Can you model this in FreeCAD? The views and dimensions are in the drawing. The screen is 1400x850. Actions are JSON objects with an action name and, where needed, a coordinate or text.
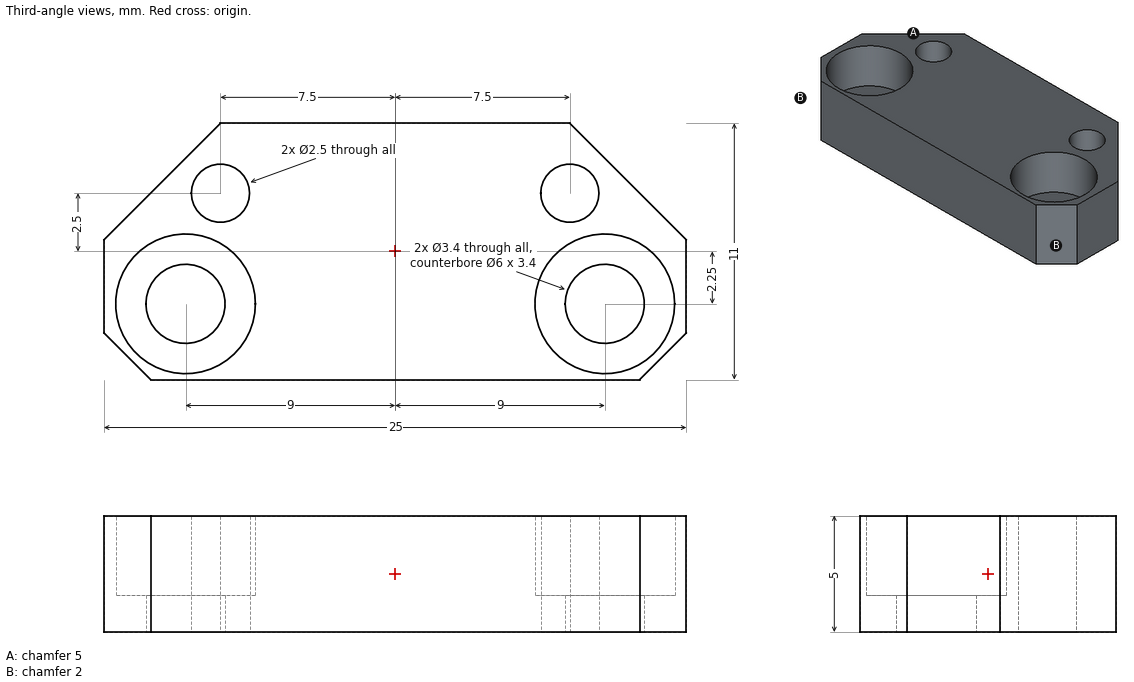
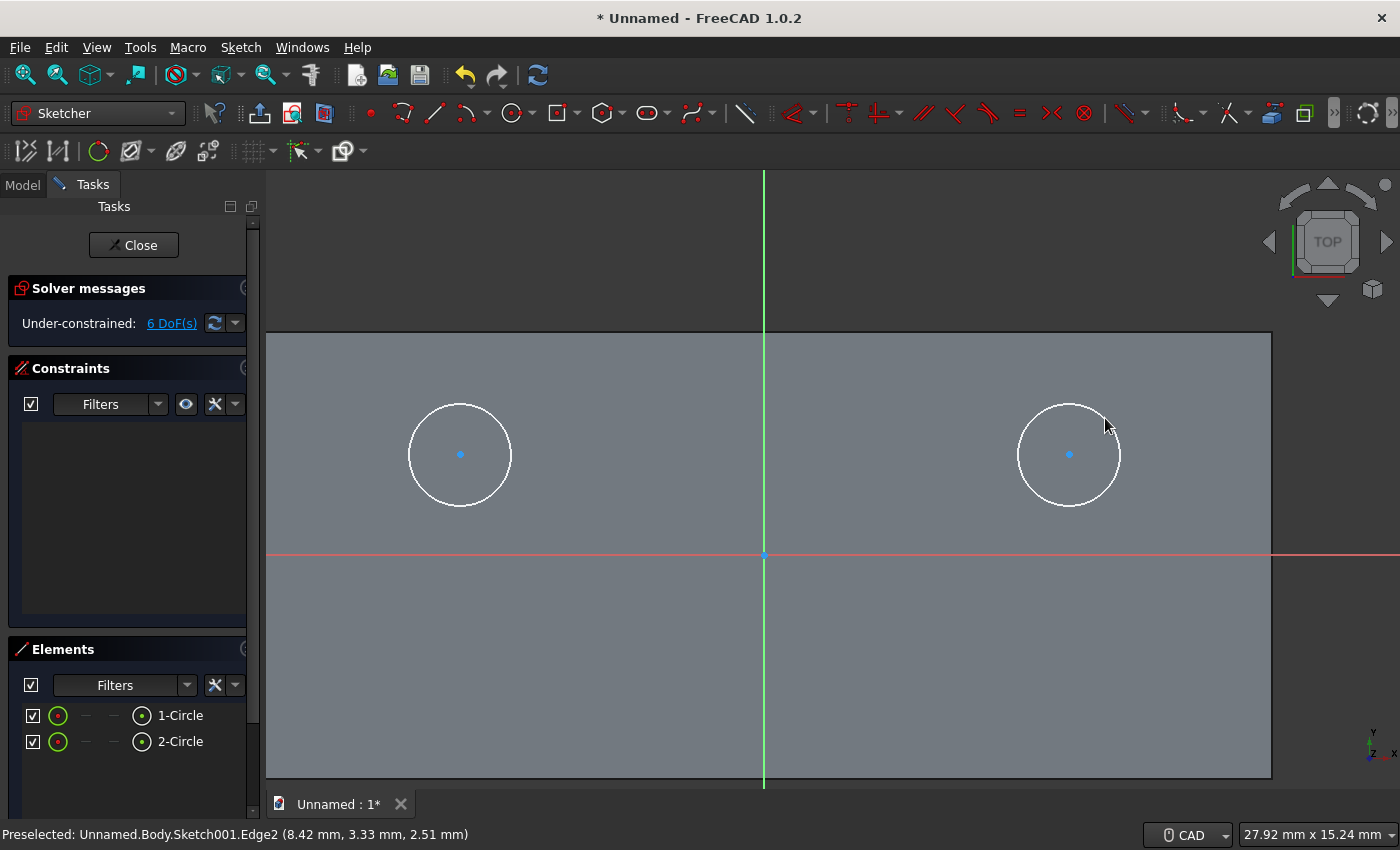
{"action": "left_click", "coordinate": [496, 419]}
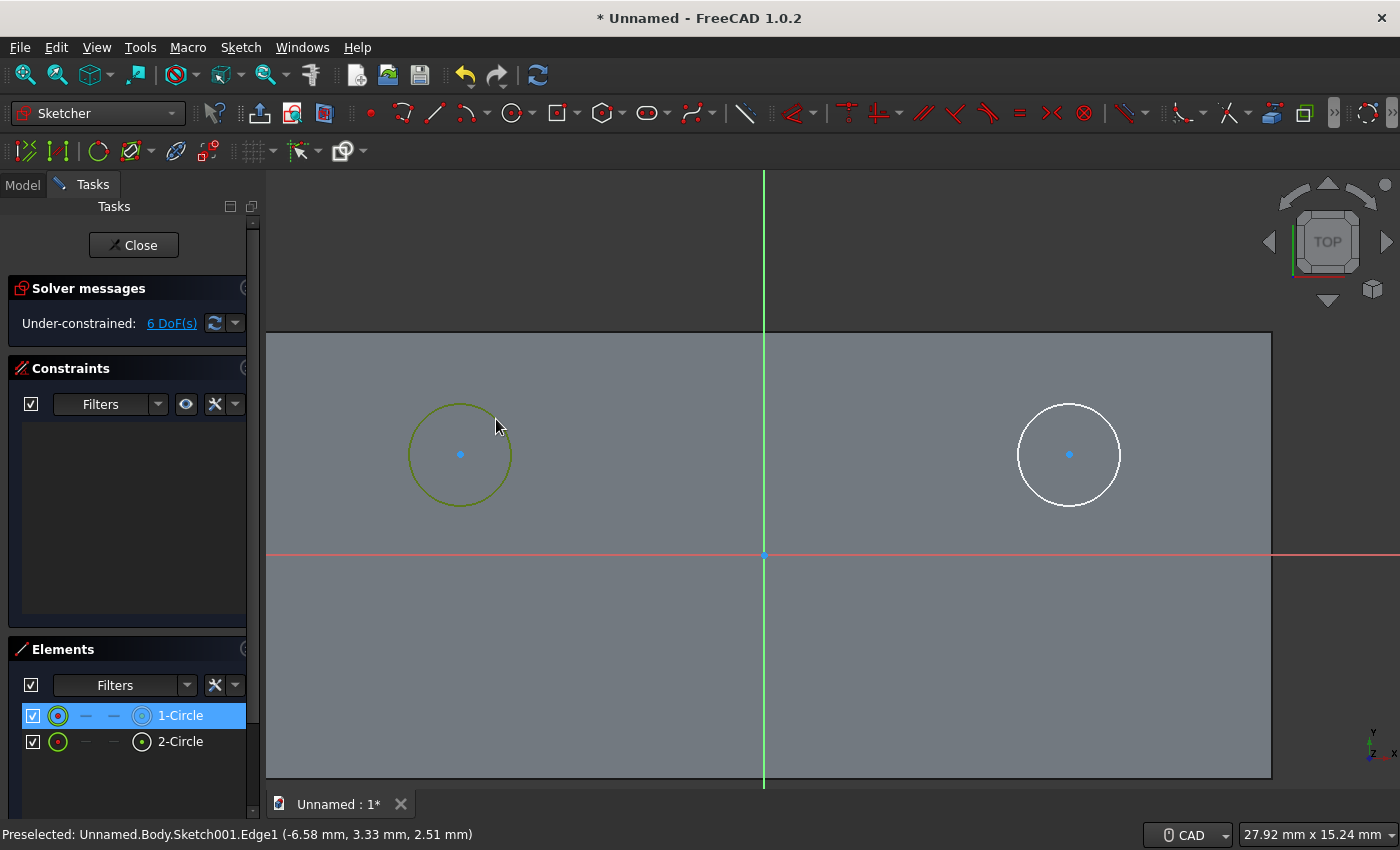
{"action": "left_click", "coordinate": [1105, 419]}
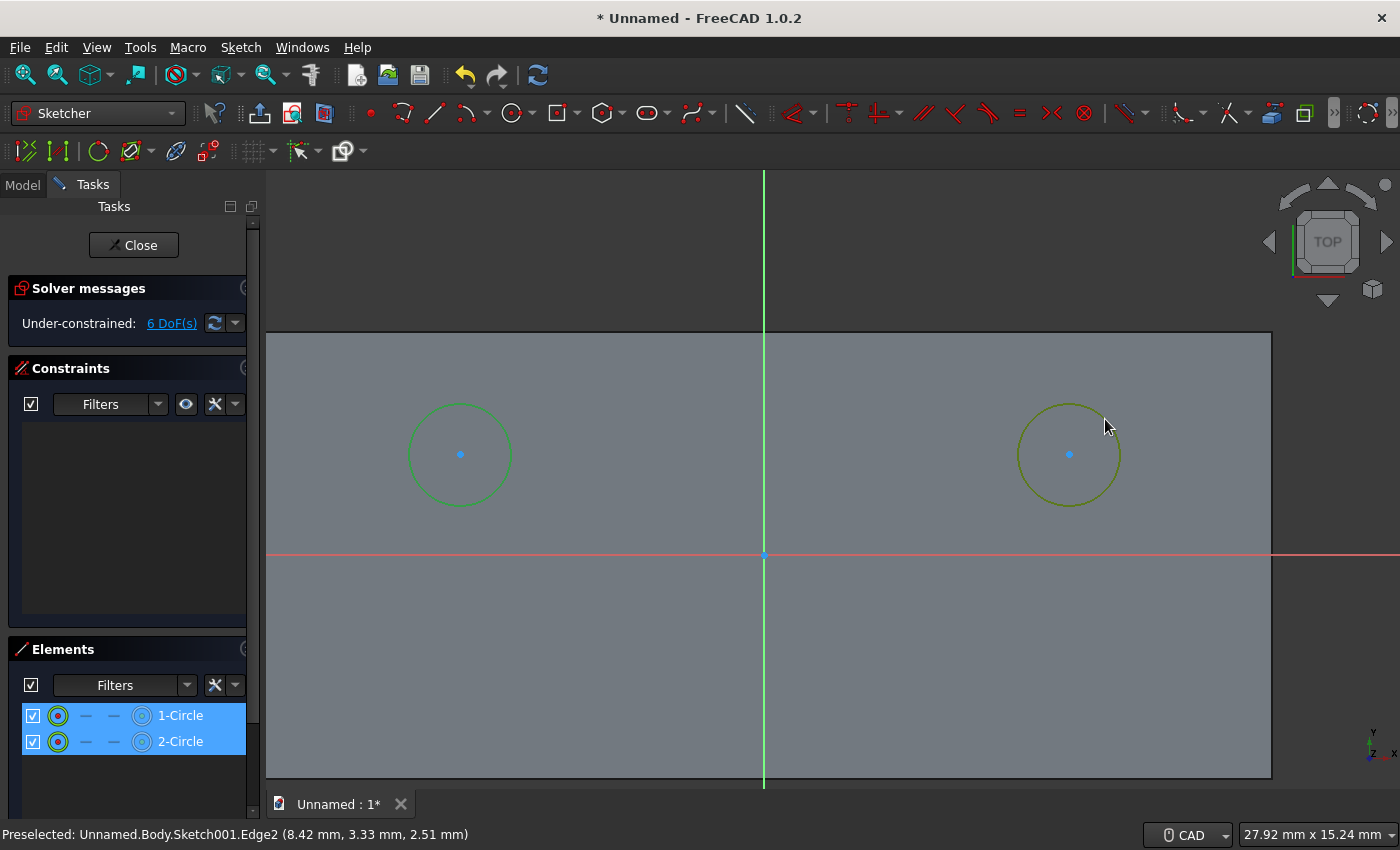
{"action": "key", "text": "e"}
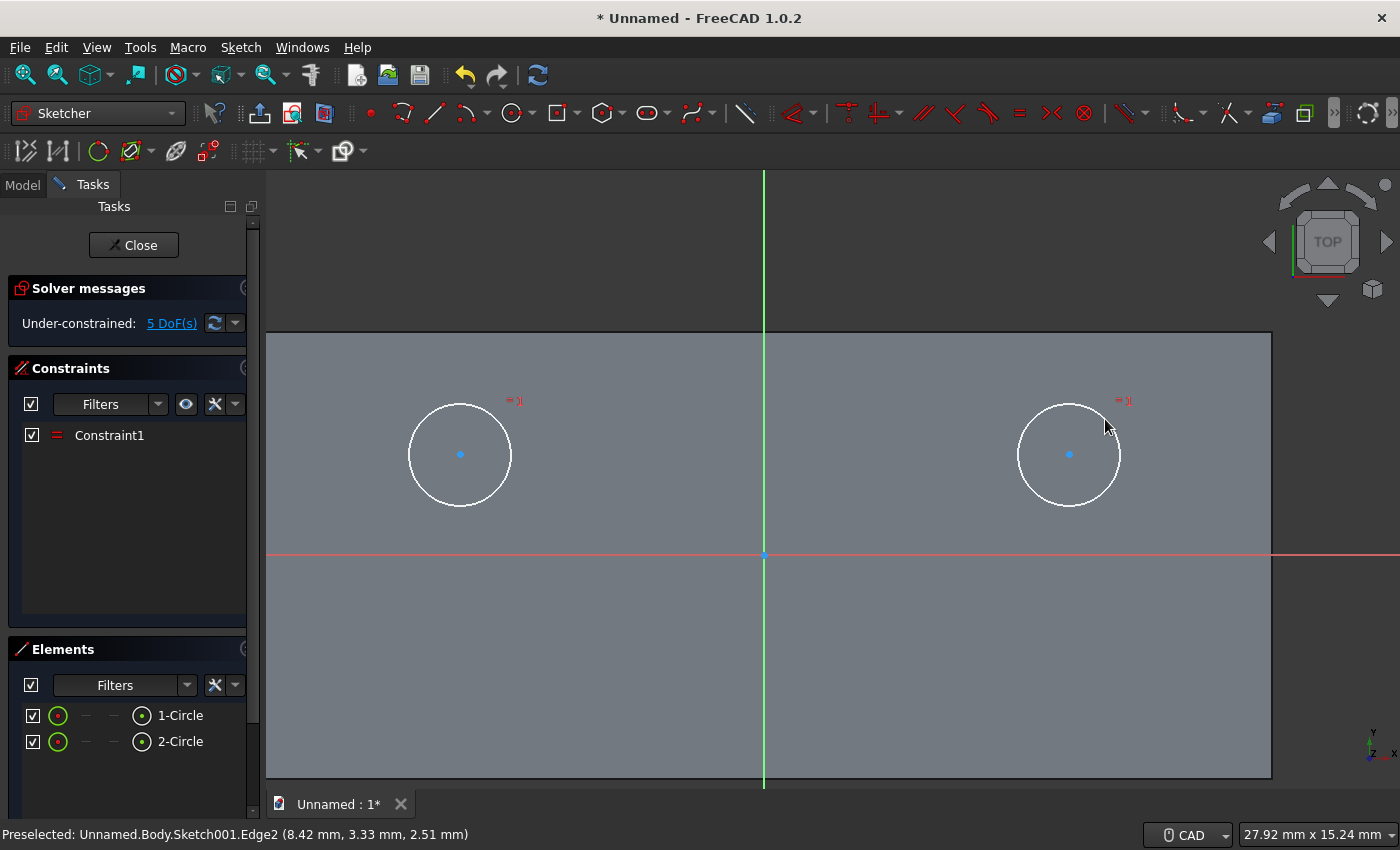
{"action": "left_click", "coordinate": [460, 455]}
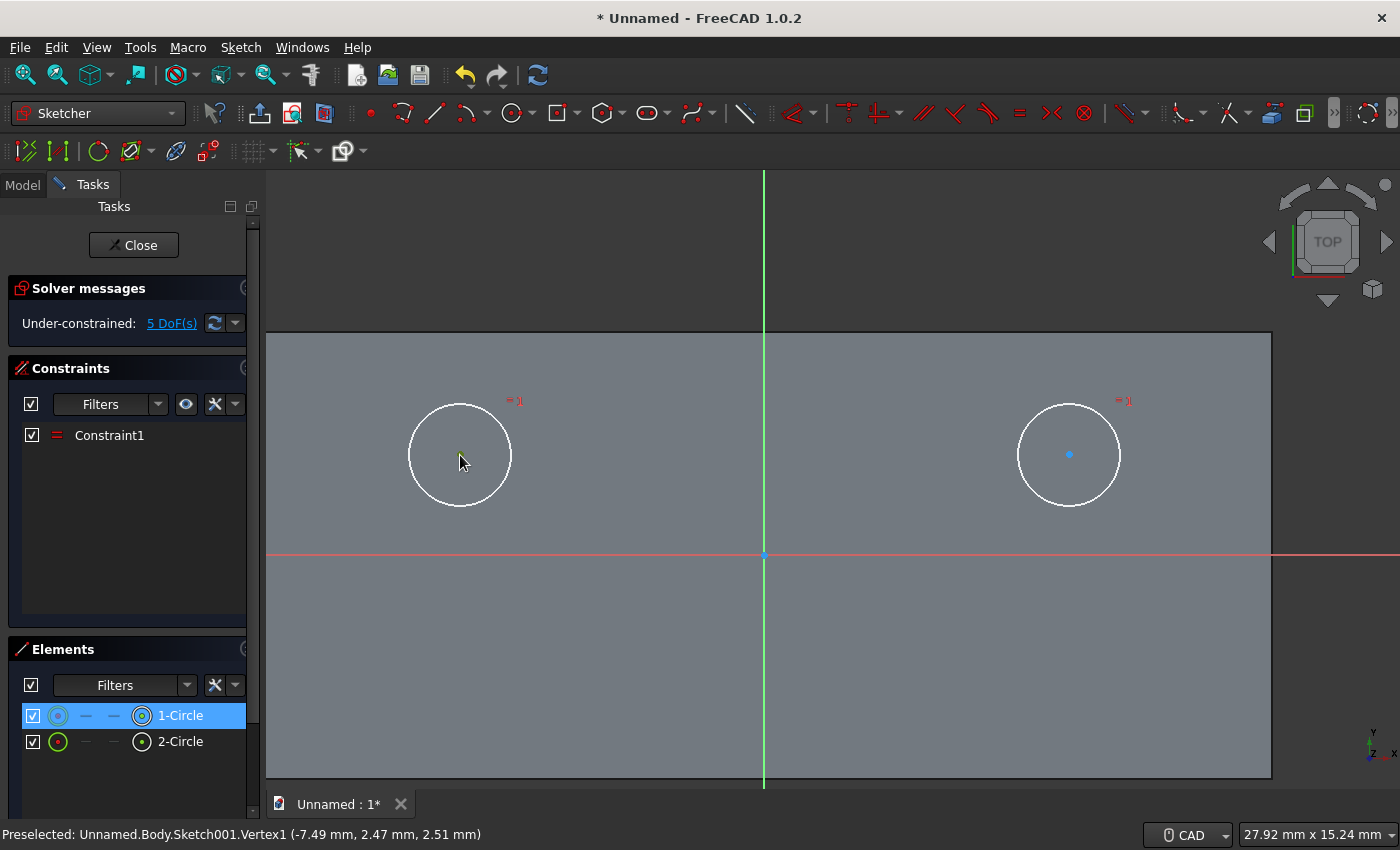
{"action": "left_click", "coordinate": [1069, 455]}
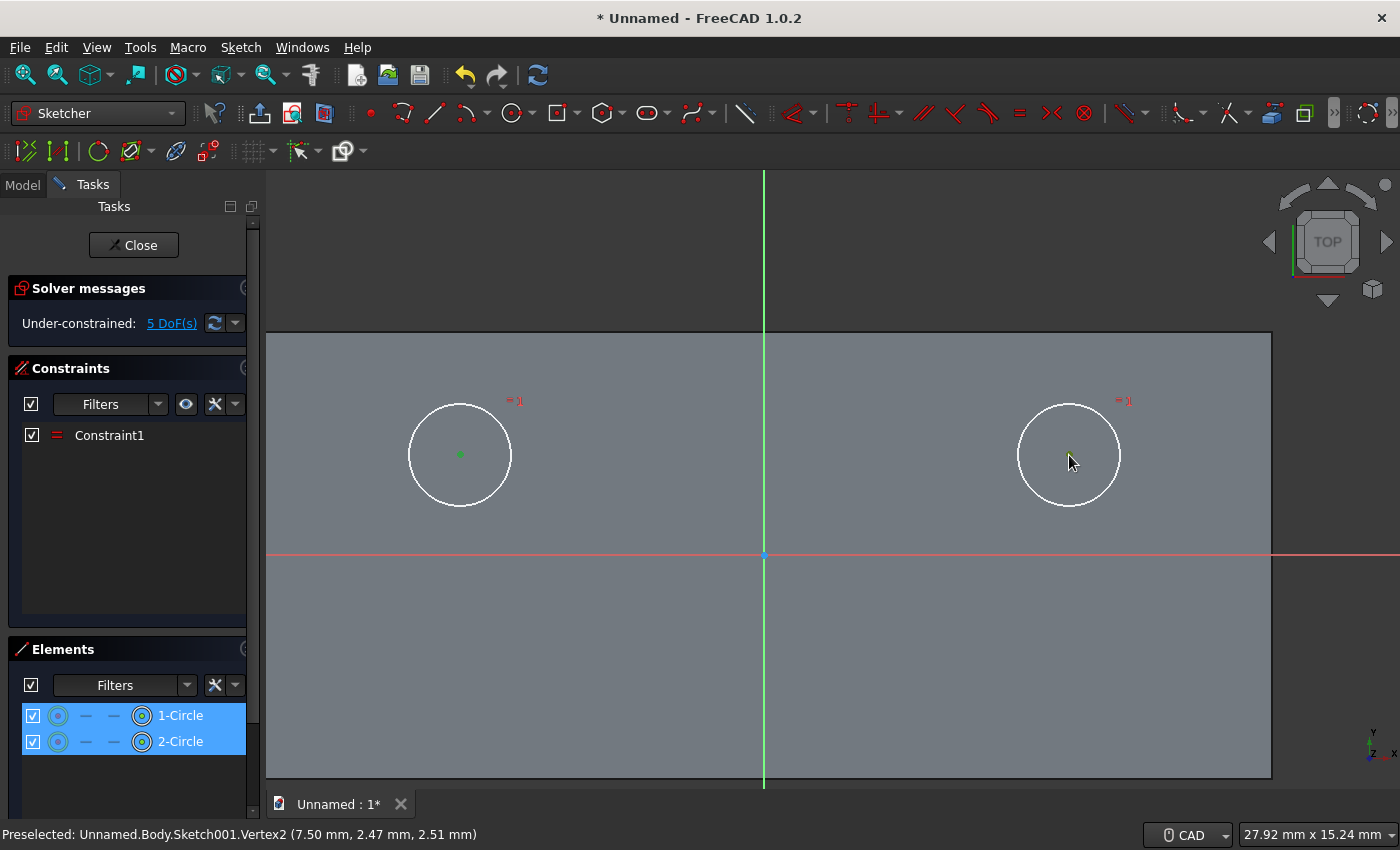
{"action": "left_click", "coordinate": [902, 114]}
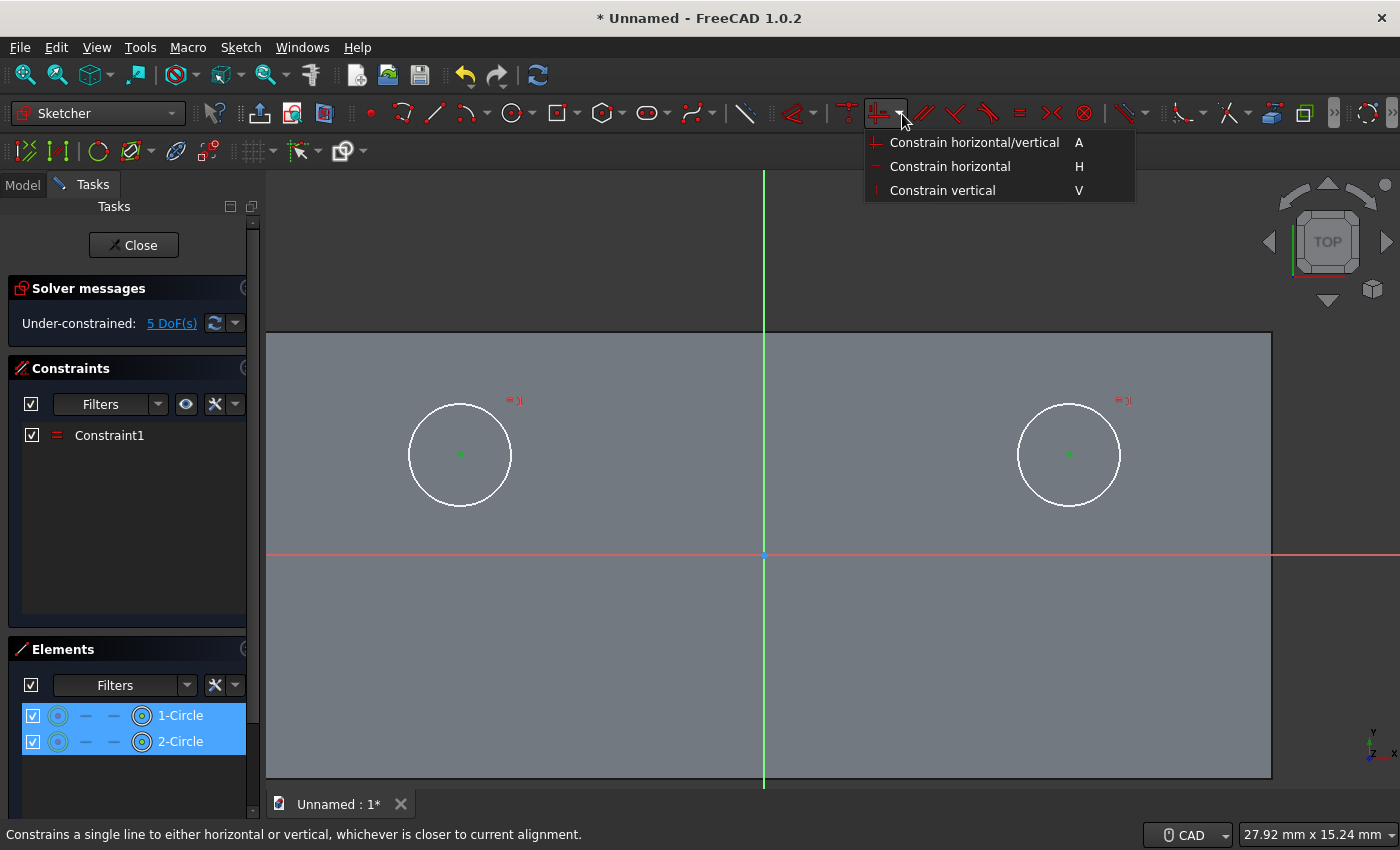
{"action": "left_click", "coordinate": [1000, 166]}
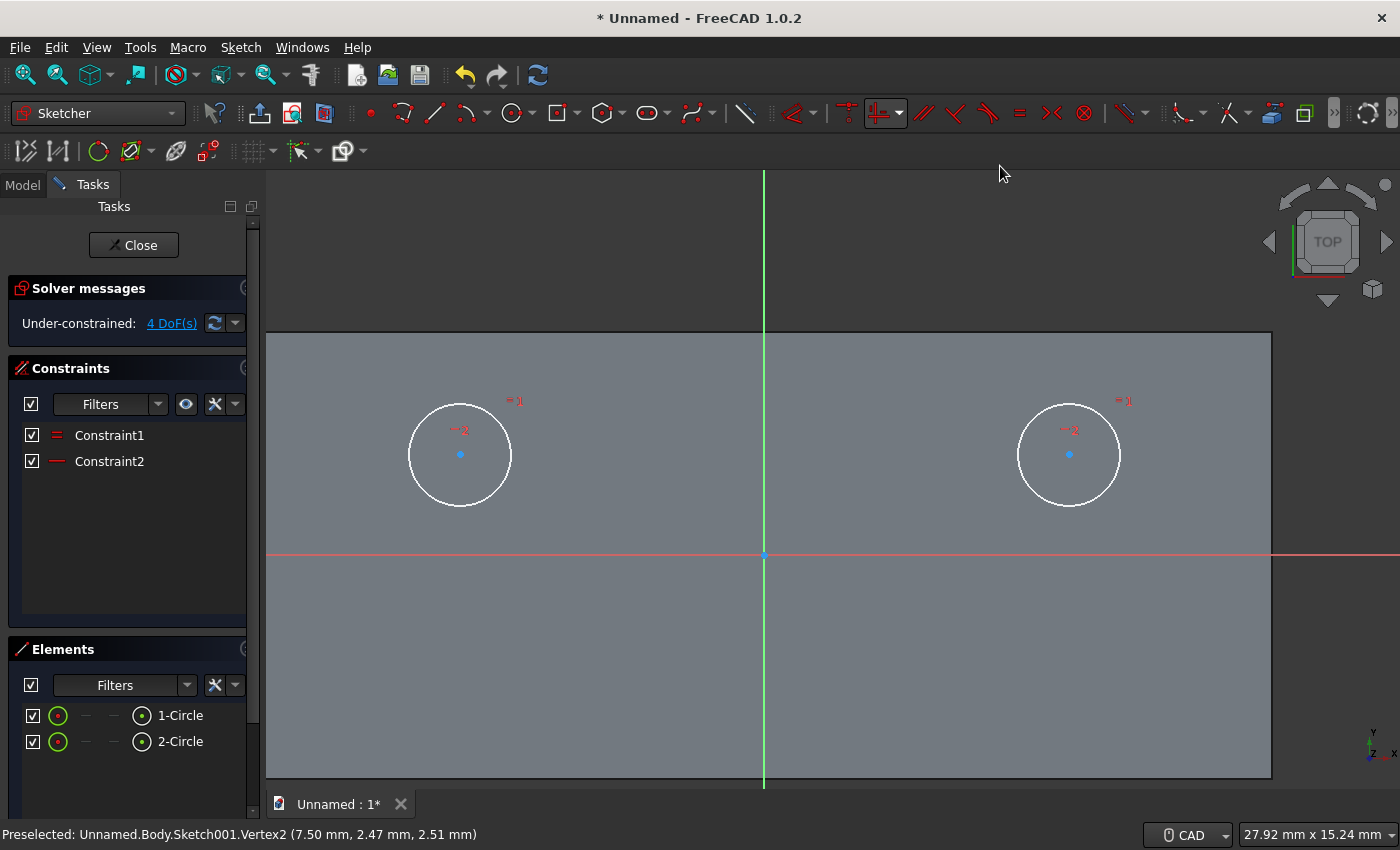
{"action": "left_click", "coordinate": [792, 114]}